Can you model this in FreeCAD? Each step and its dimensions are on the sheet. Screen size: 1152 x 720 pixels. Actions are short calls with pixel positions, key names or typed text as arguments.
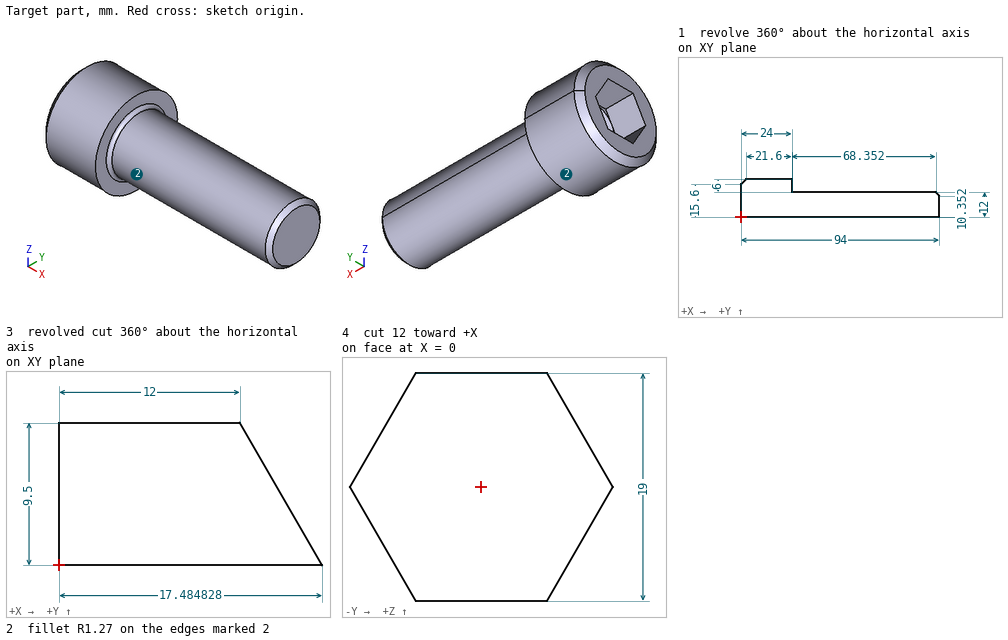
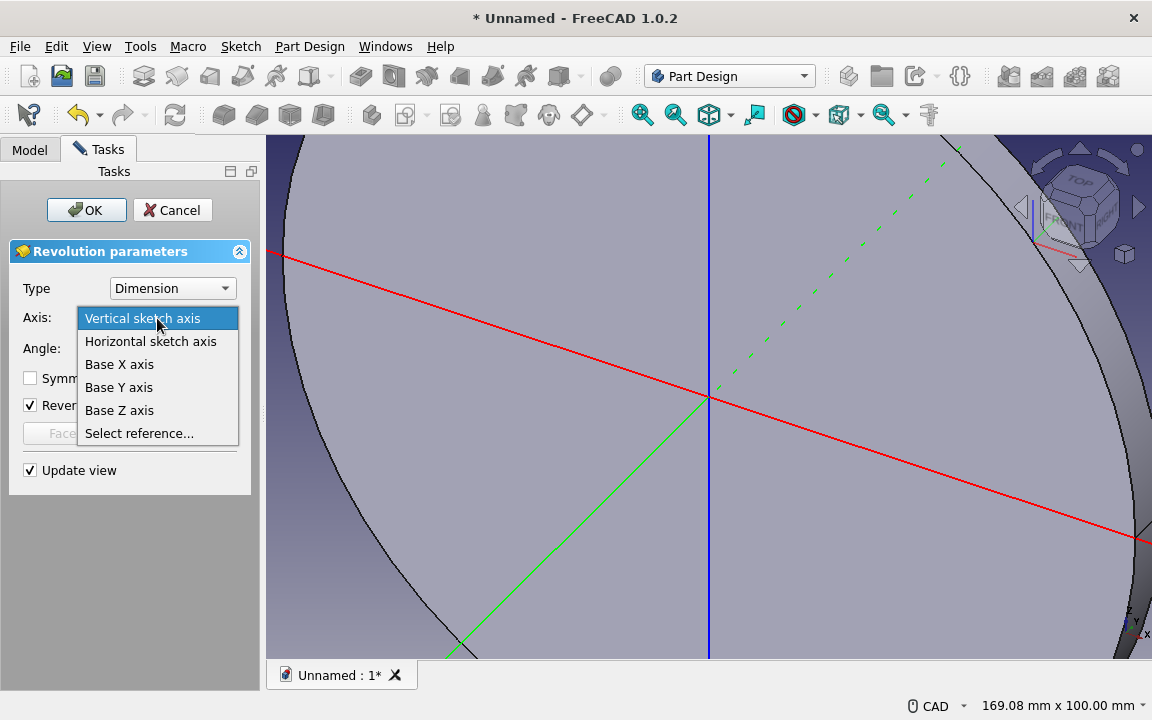
click(156, 342)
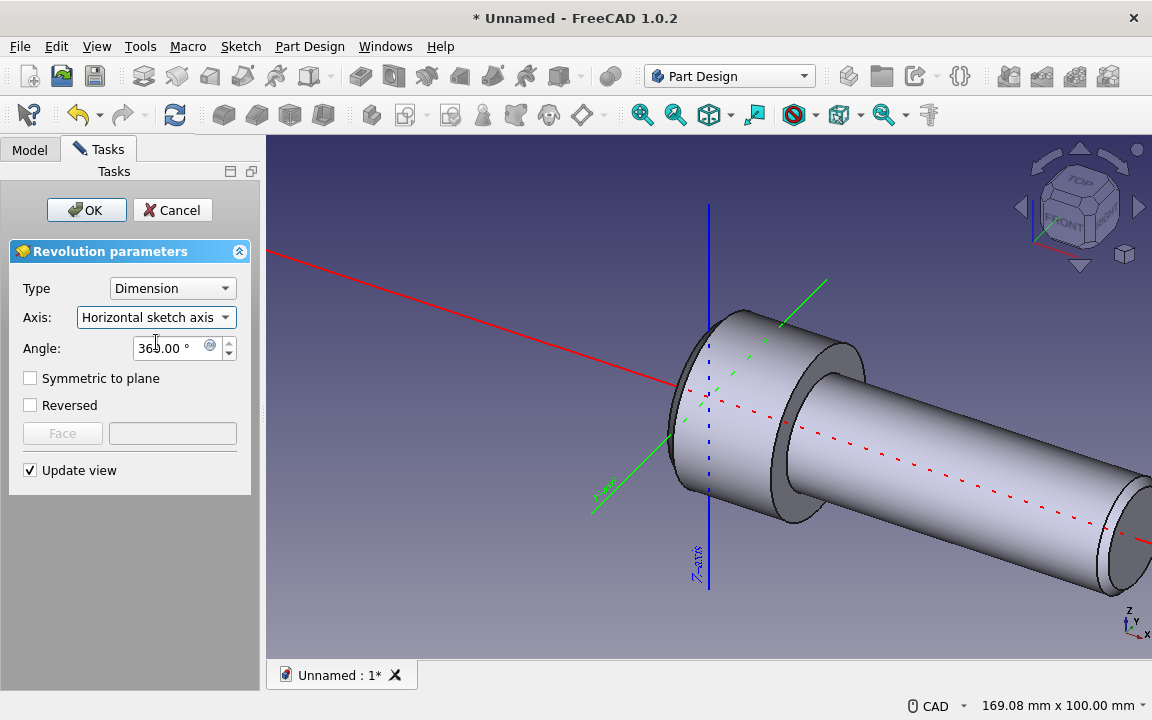
click(87, 210)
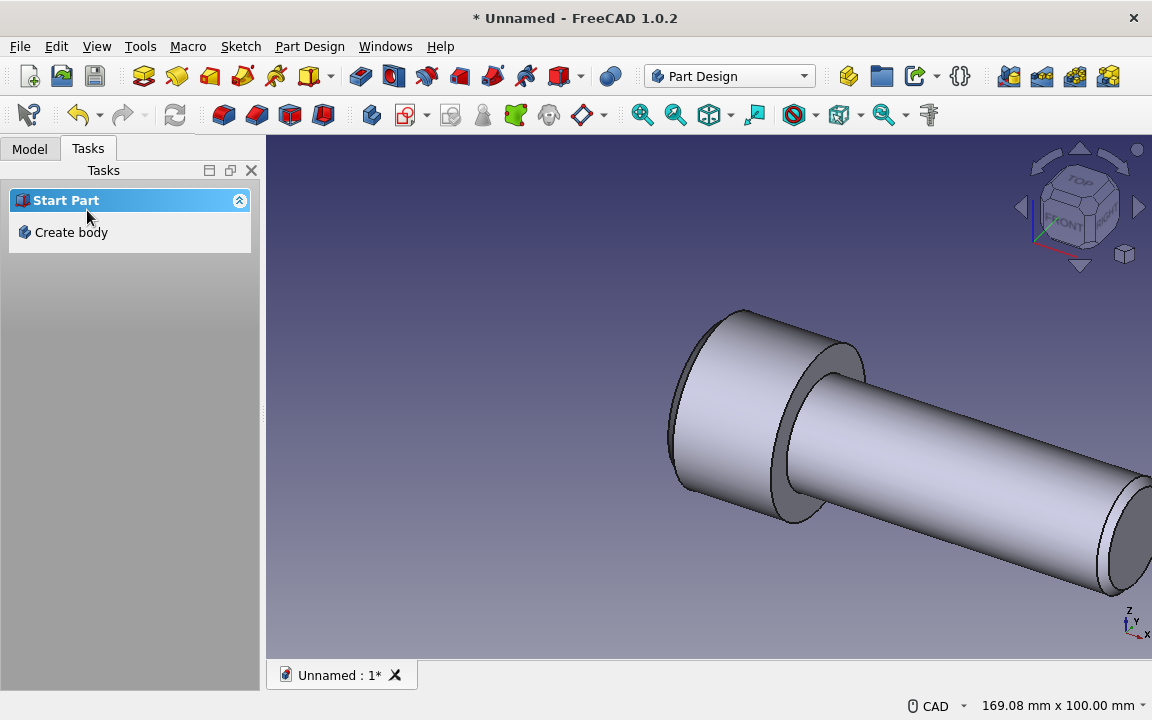
click(643, 116)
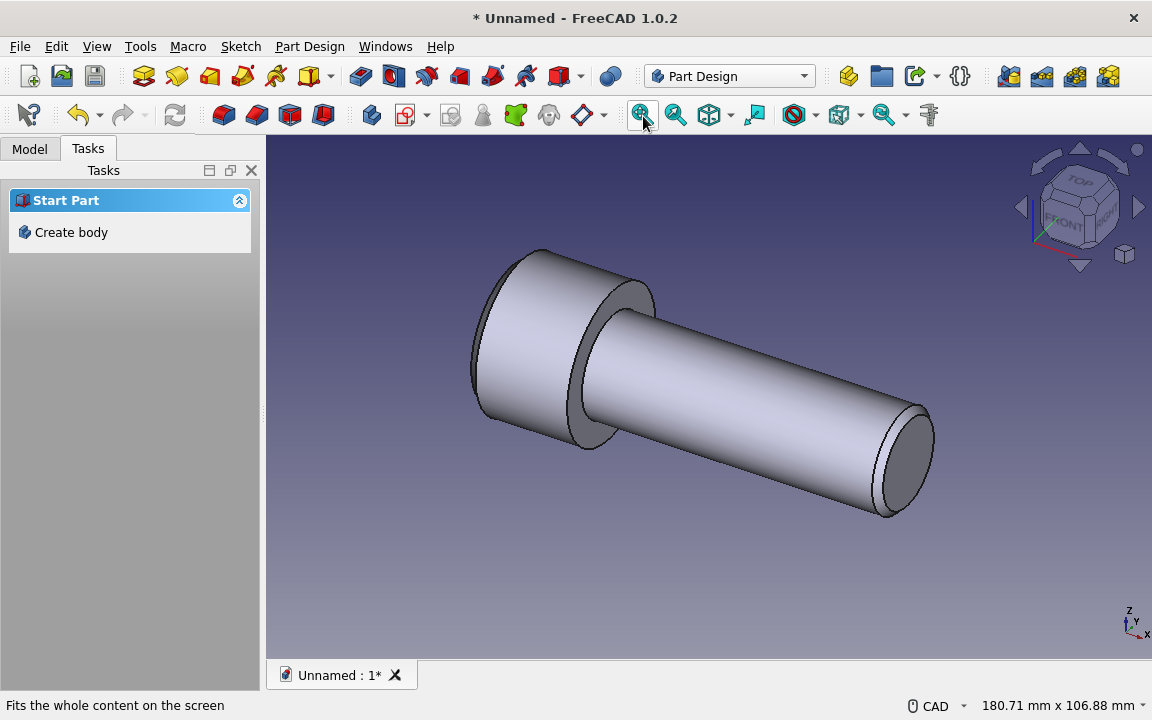
key(0)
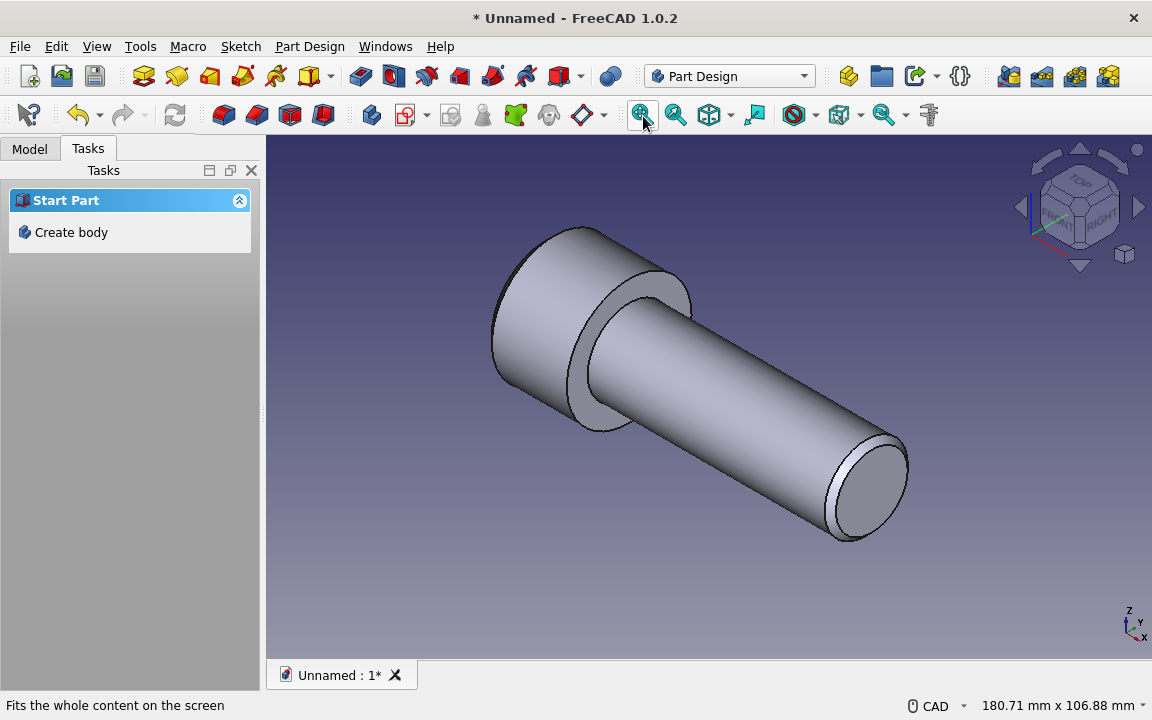
key(2)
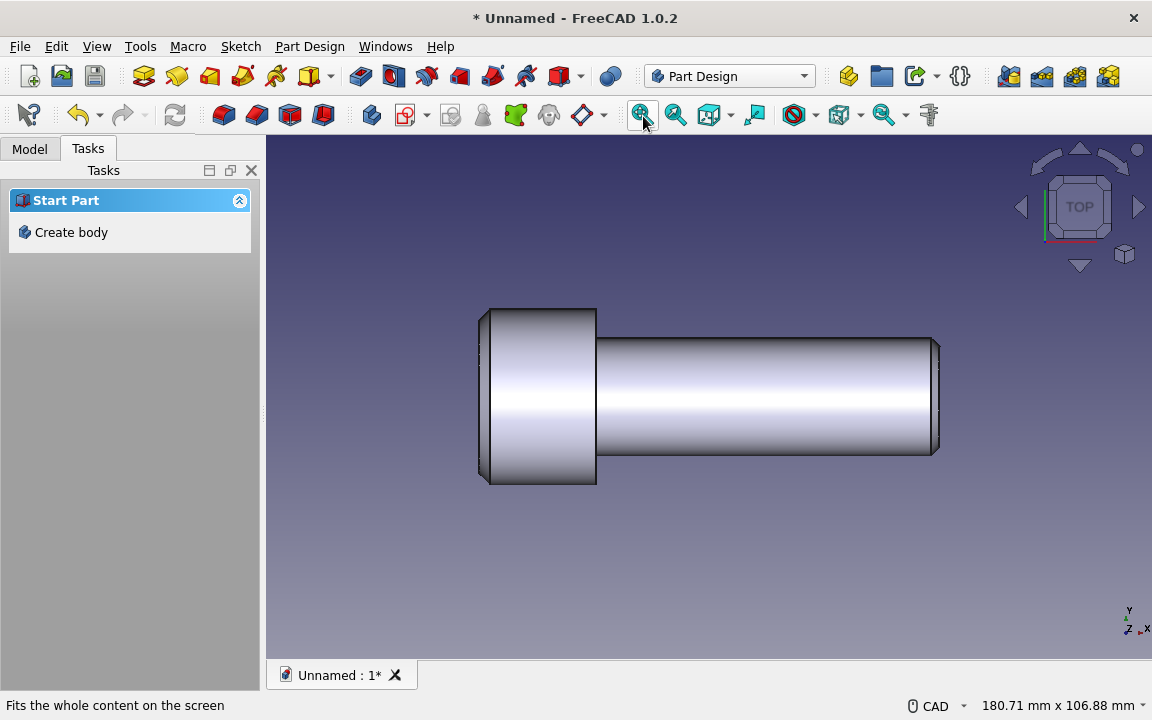
key(1)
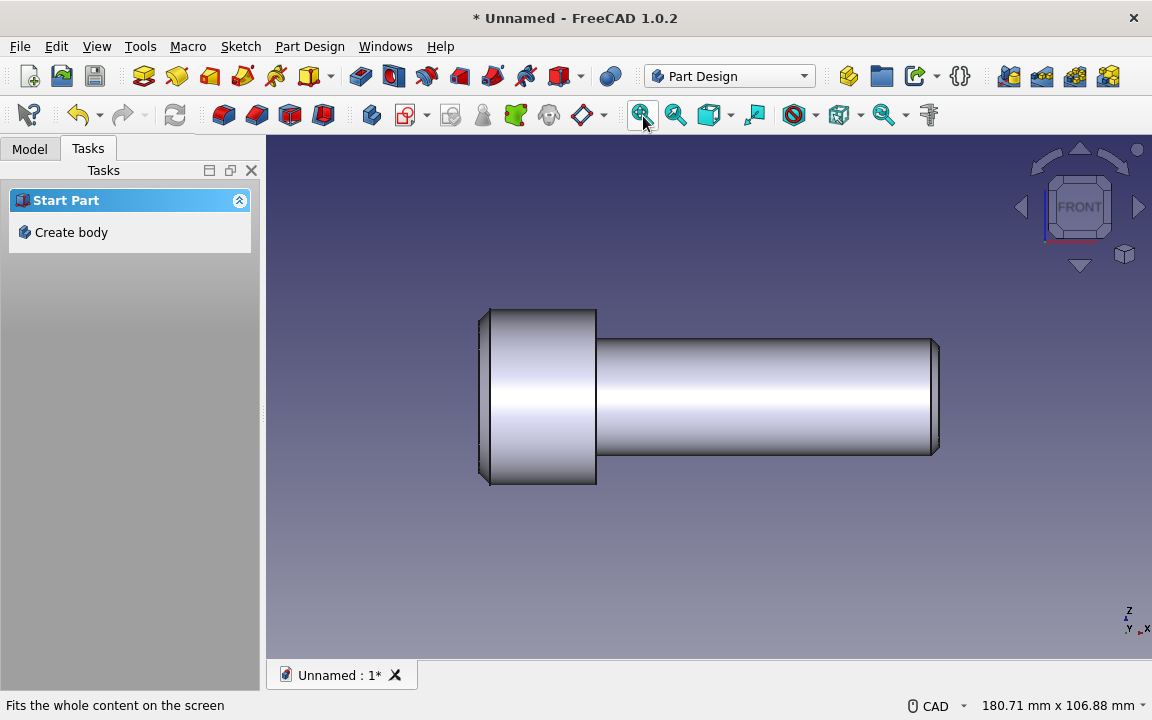
key(3)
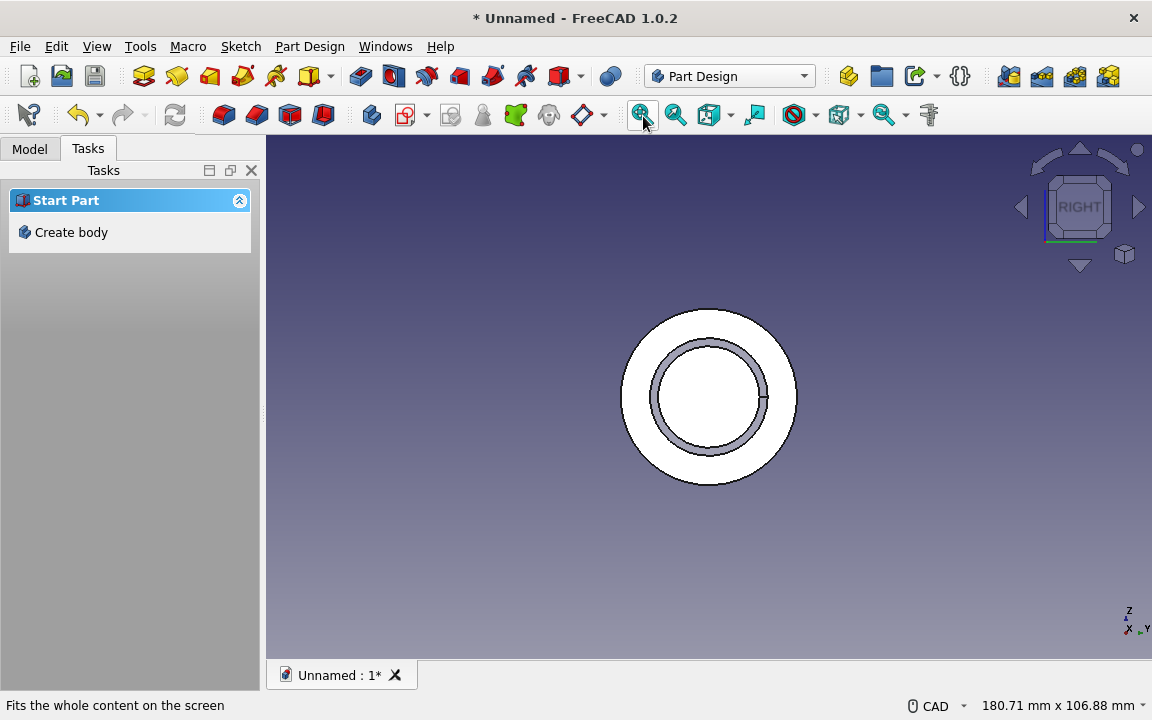
click(643, 116)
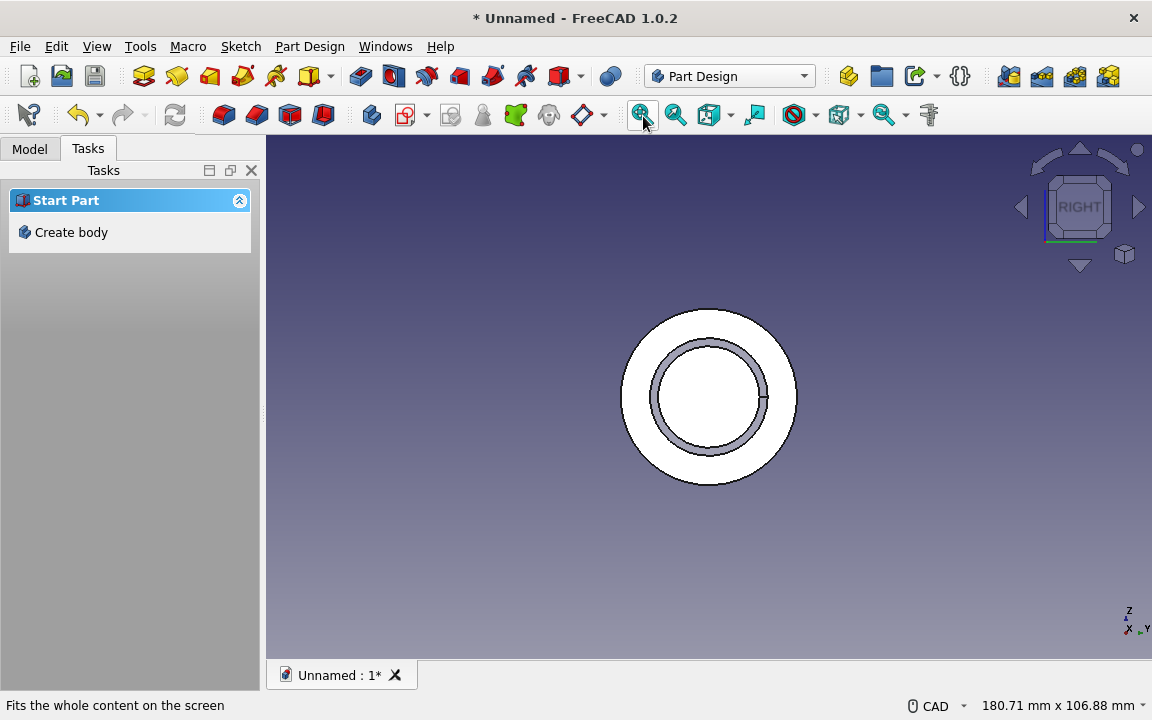
key(5)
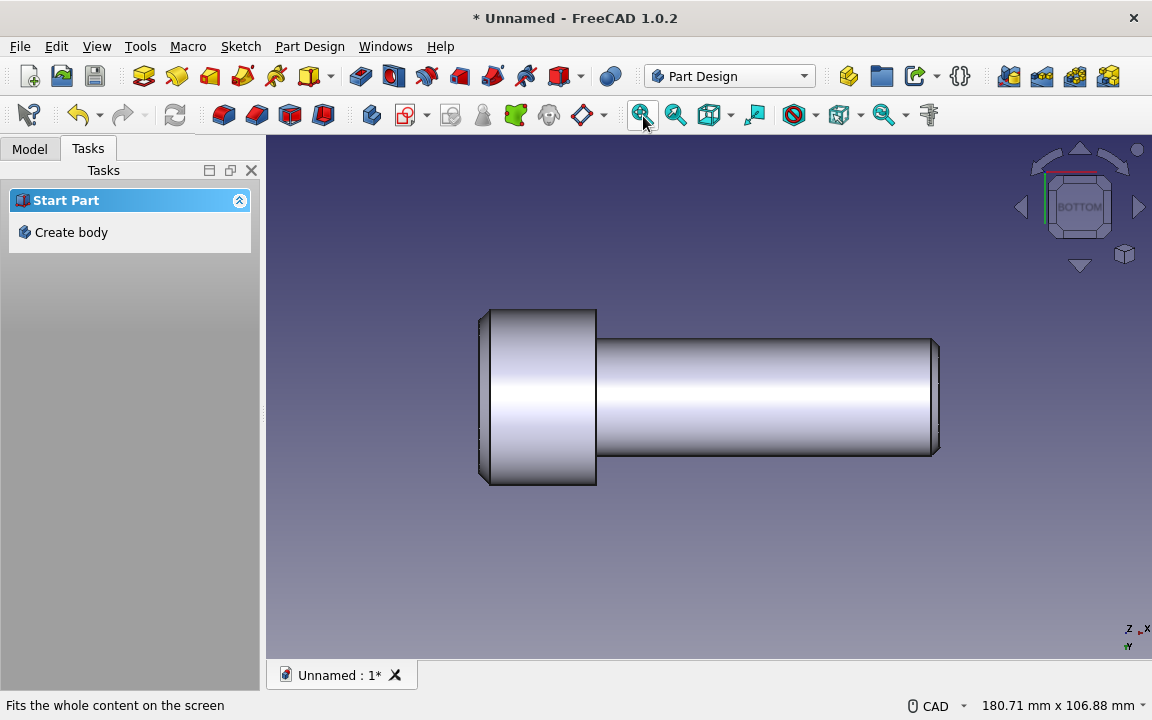
key(4)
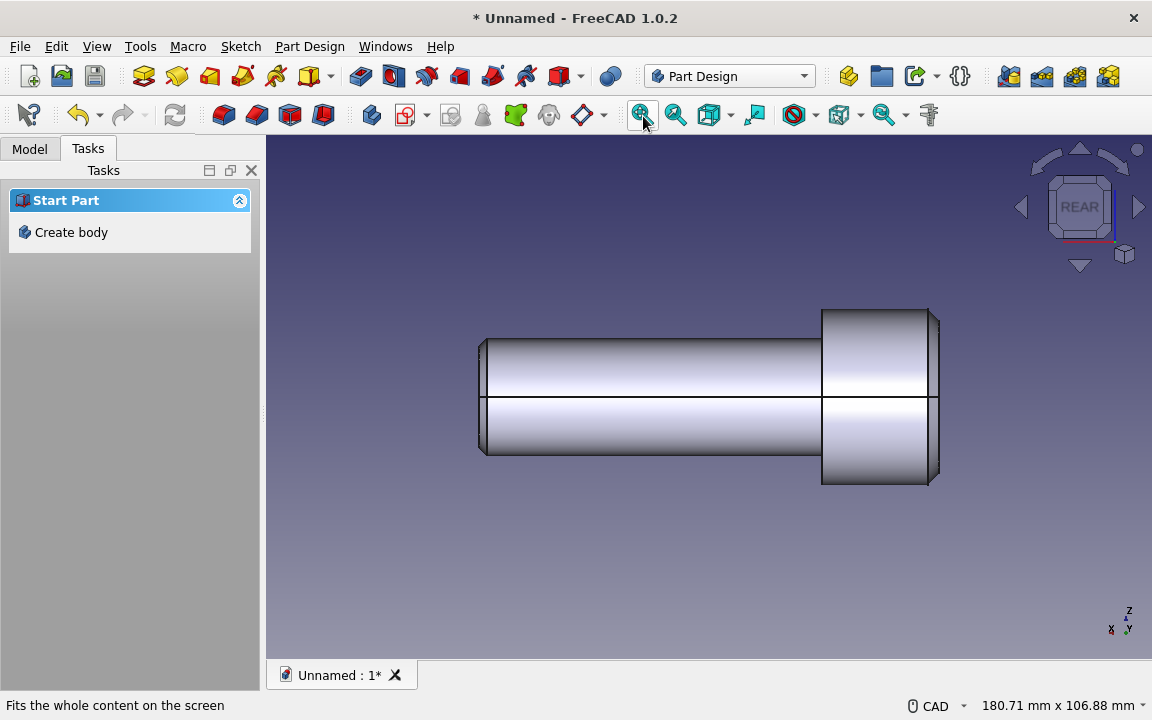
key(6)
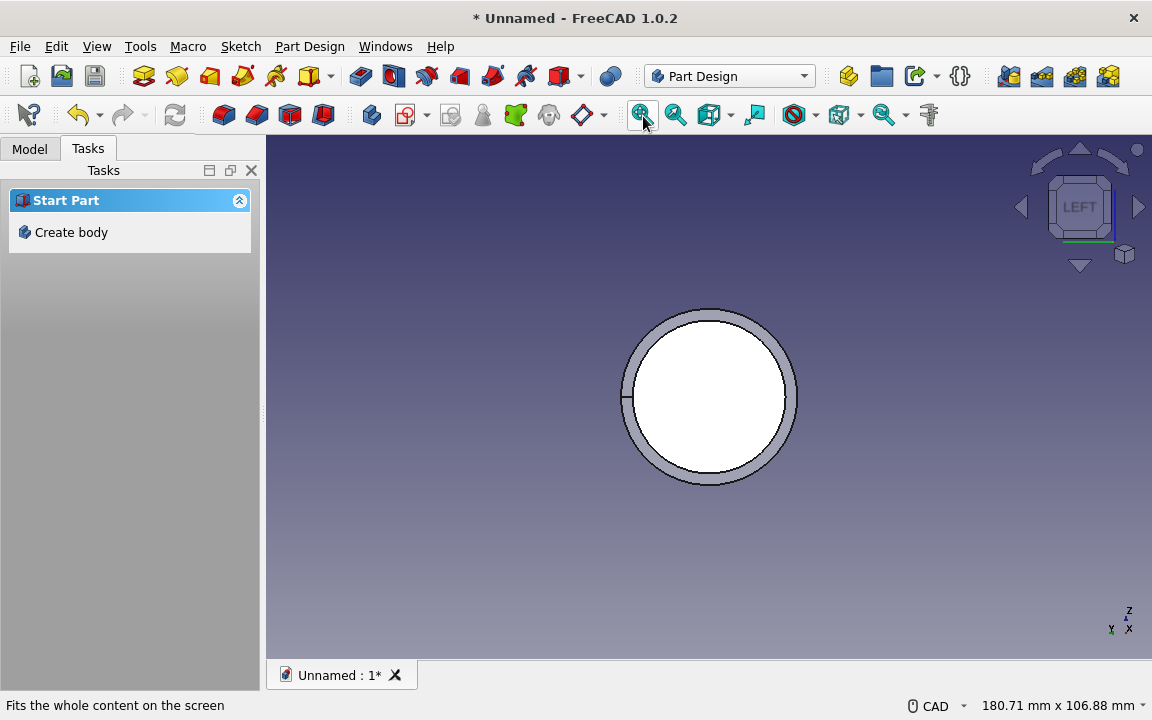
click(643, 116)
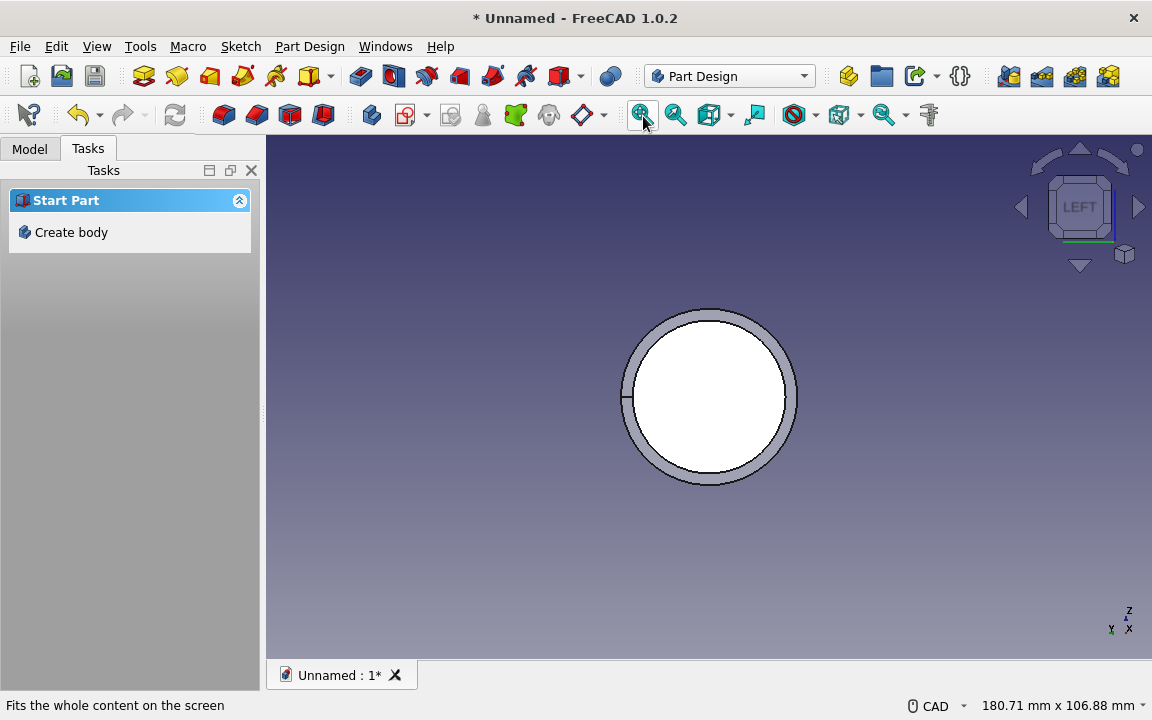
key(v)
key(3)